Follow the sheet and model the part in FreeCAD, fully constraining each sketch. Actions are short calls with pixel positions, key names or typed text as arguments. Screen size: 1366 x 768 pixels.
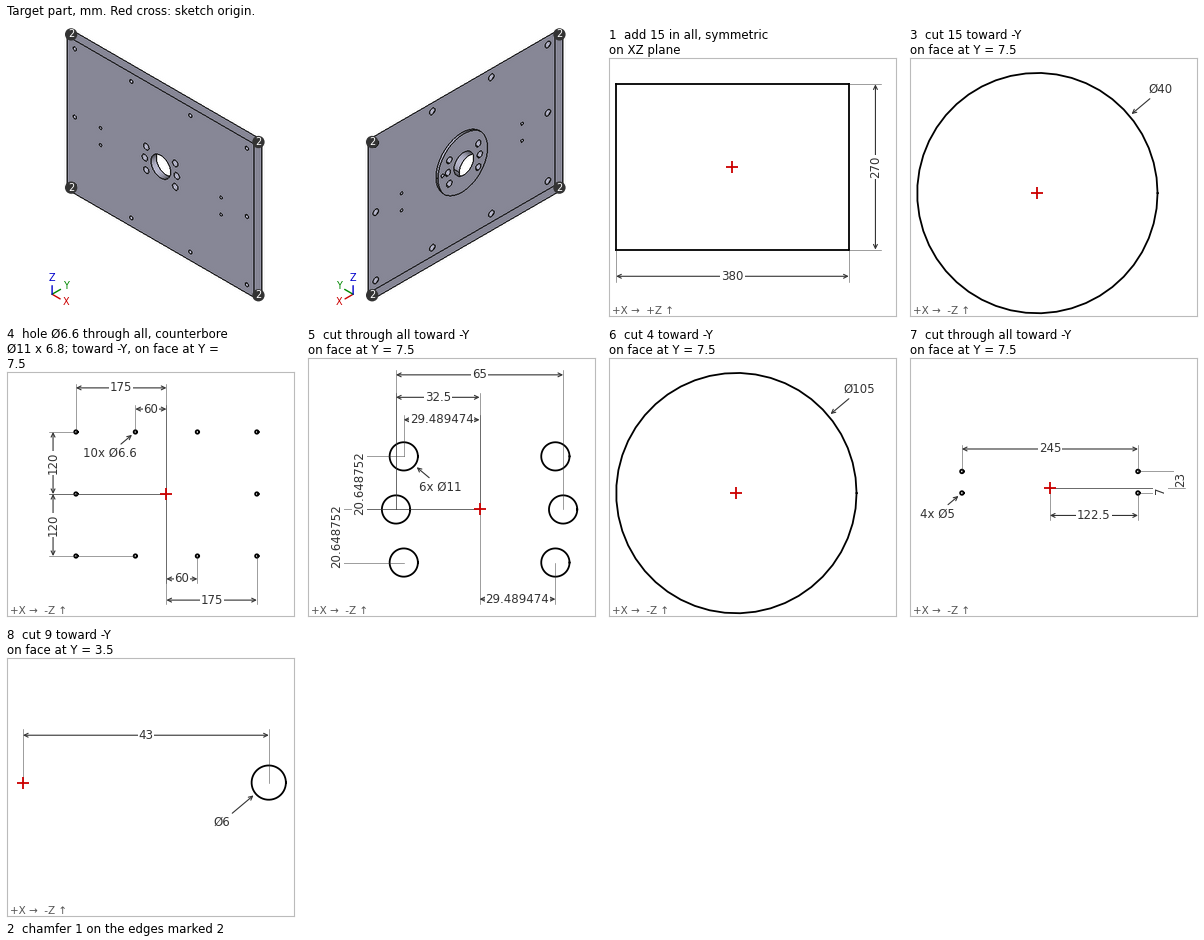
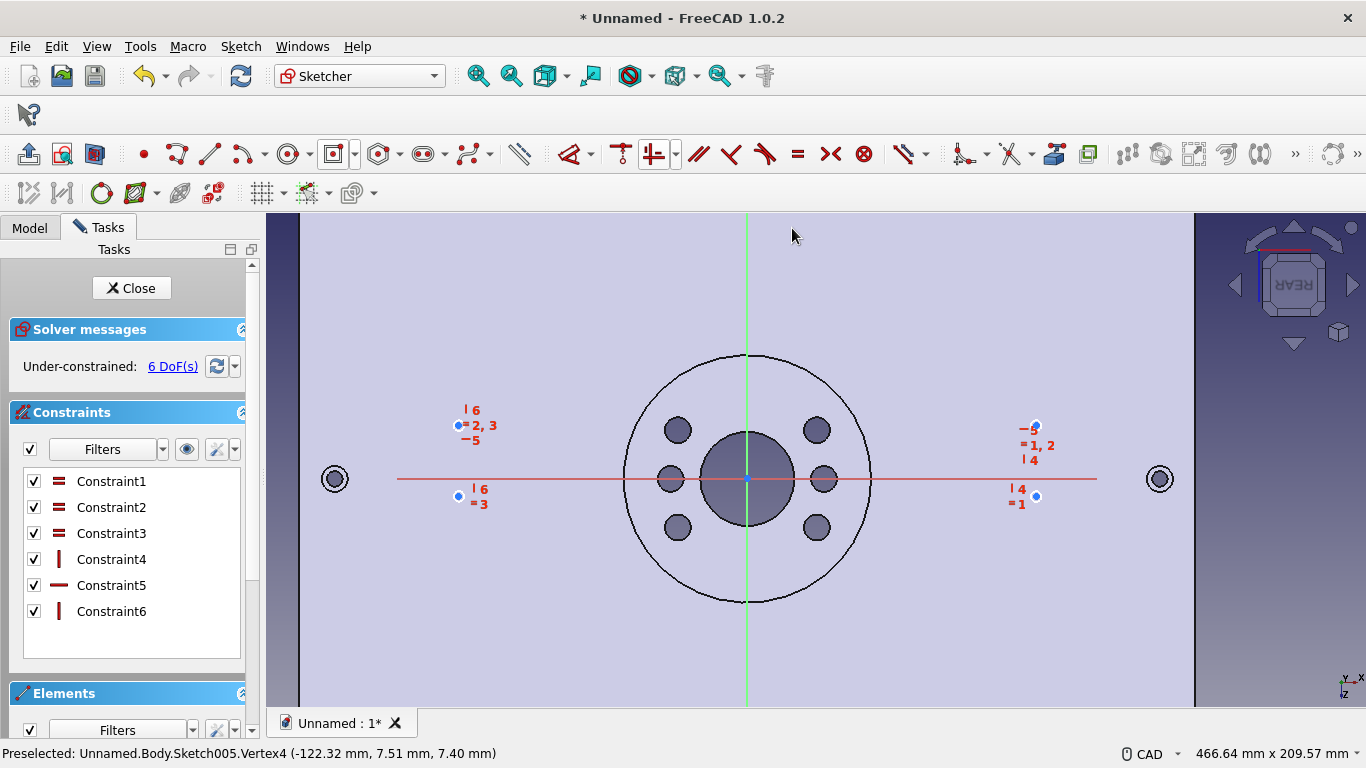
click(1036, 497)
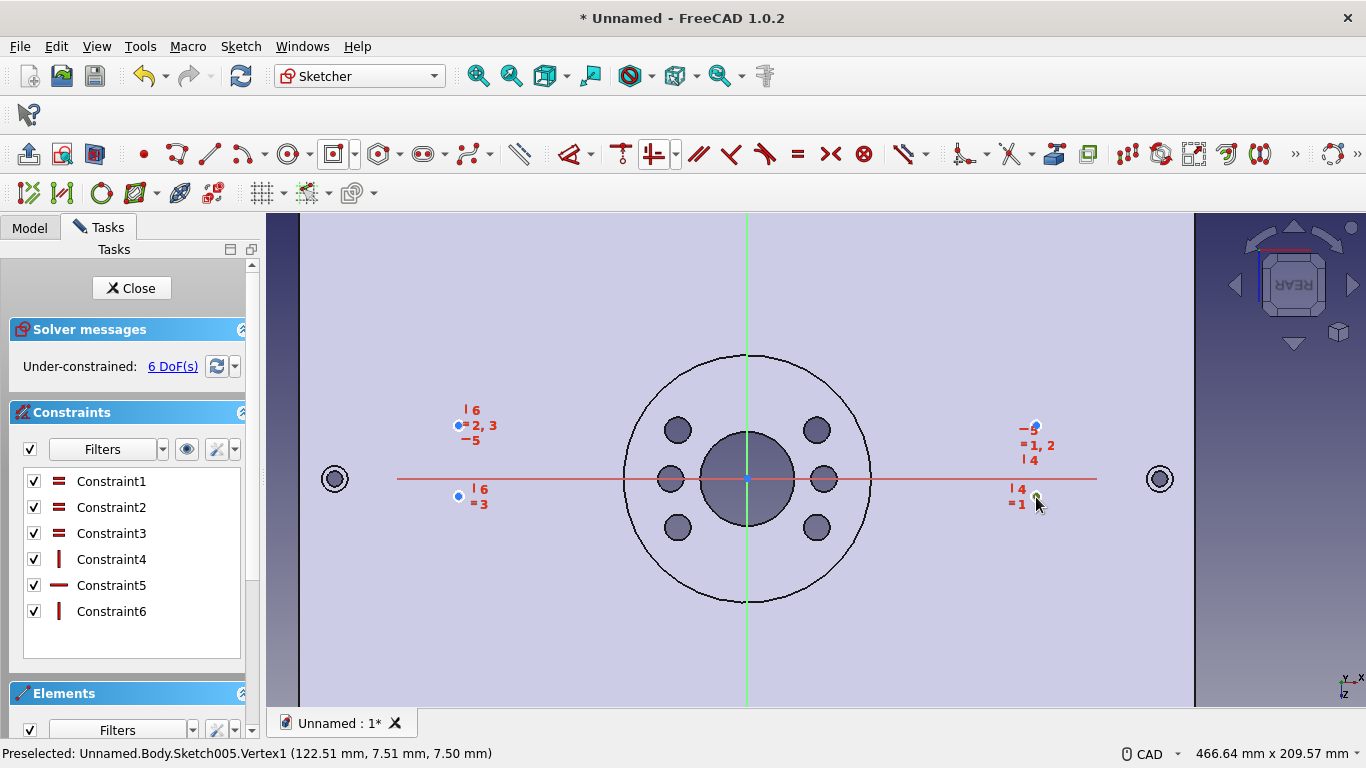
click(459, 496)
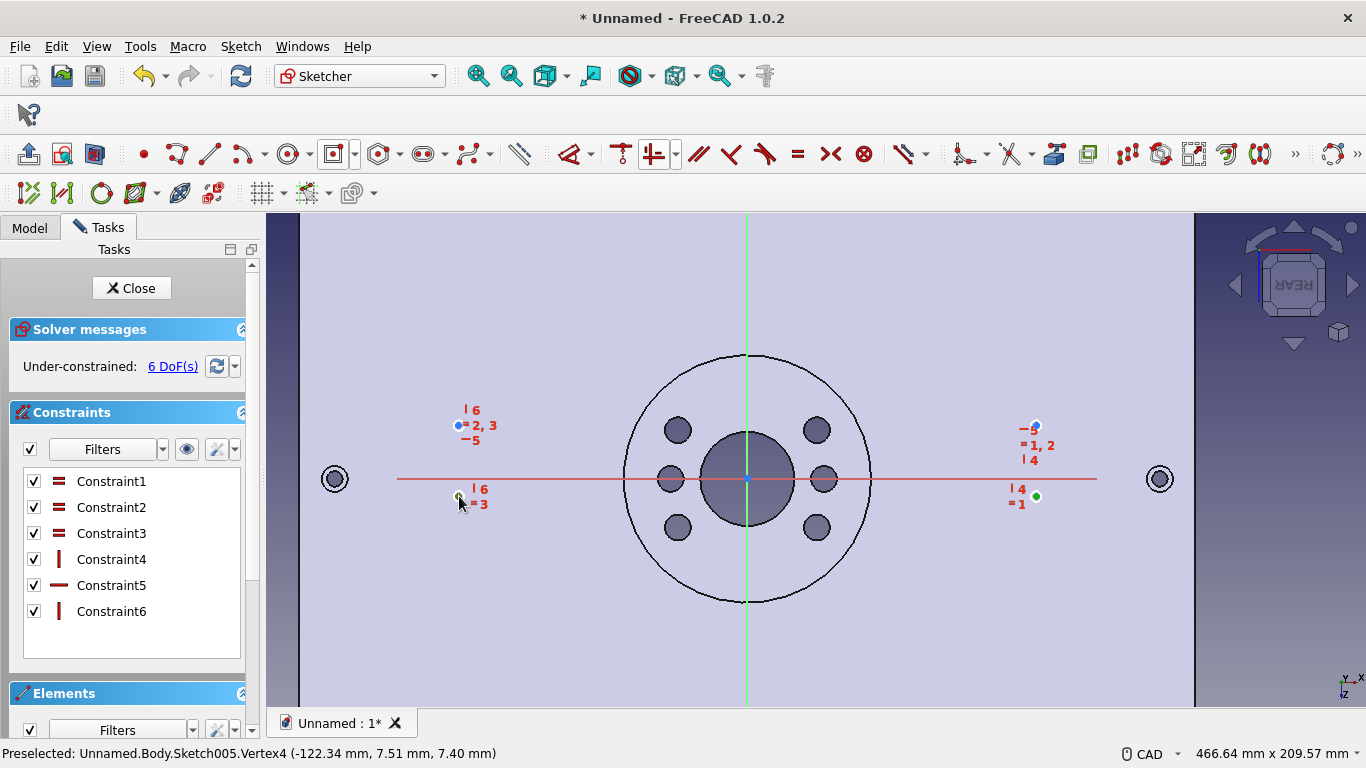
key(h)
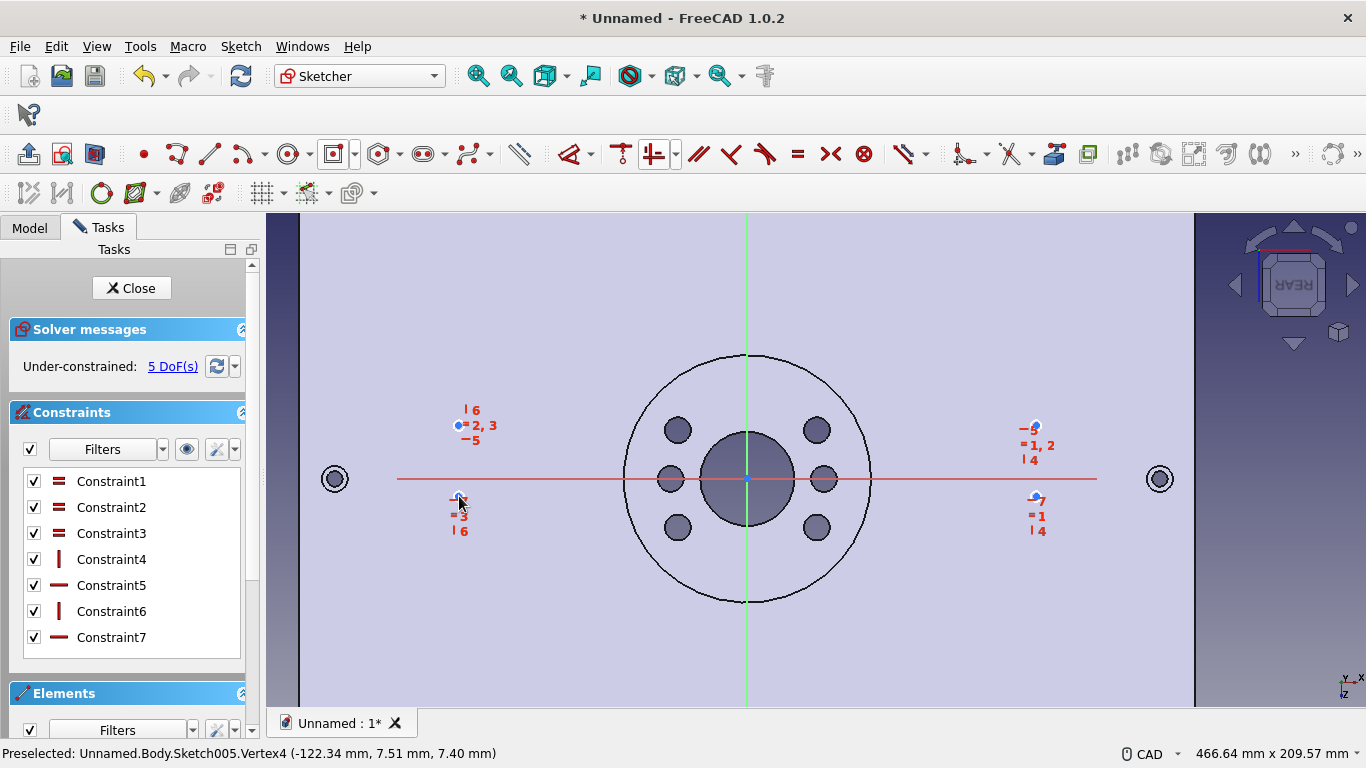
click(568, 154)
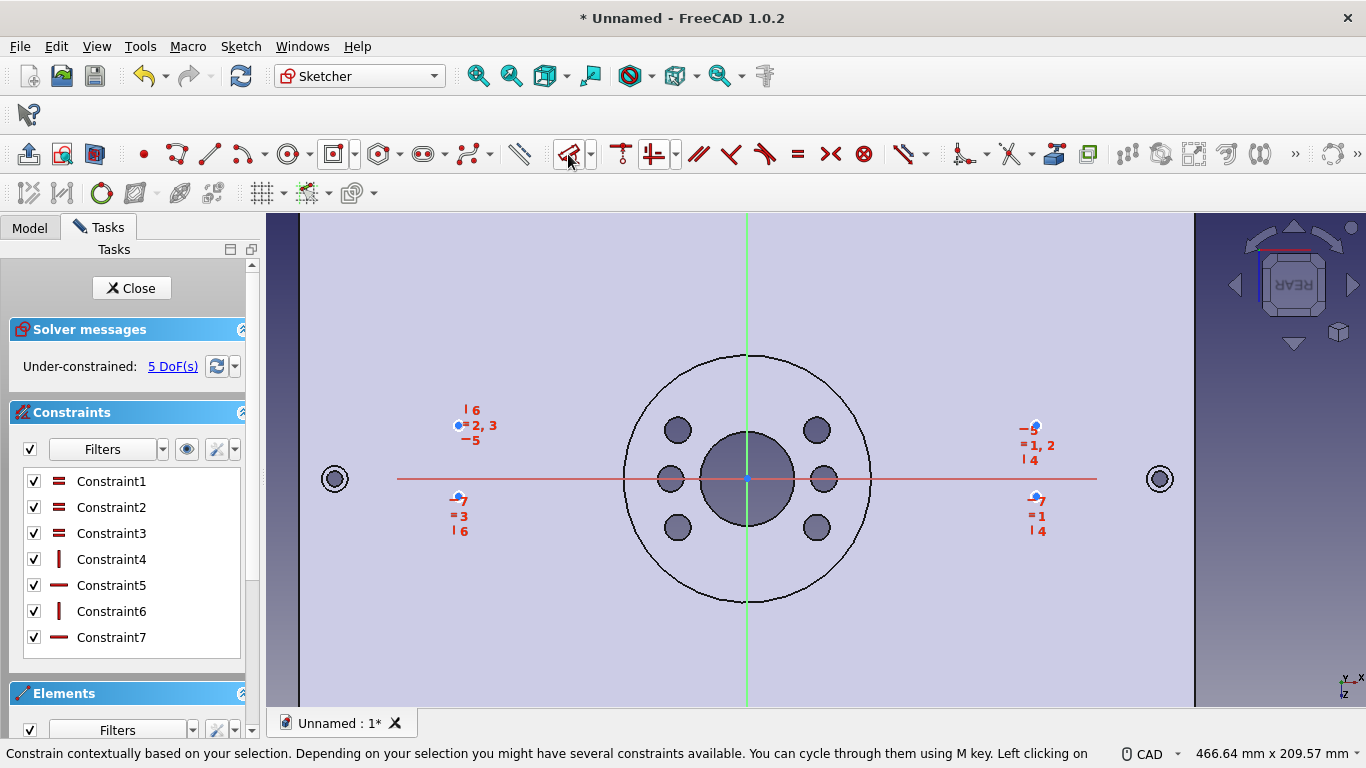
scroll(1032, 500, up, 7)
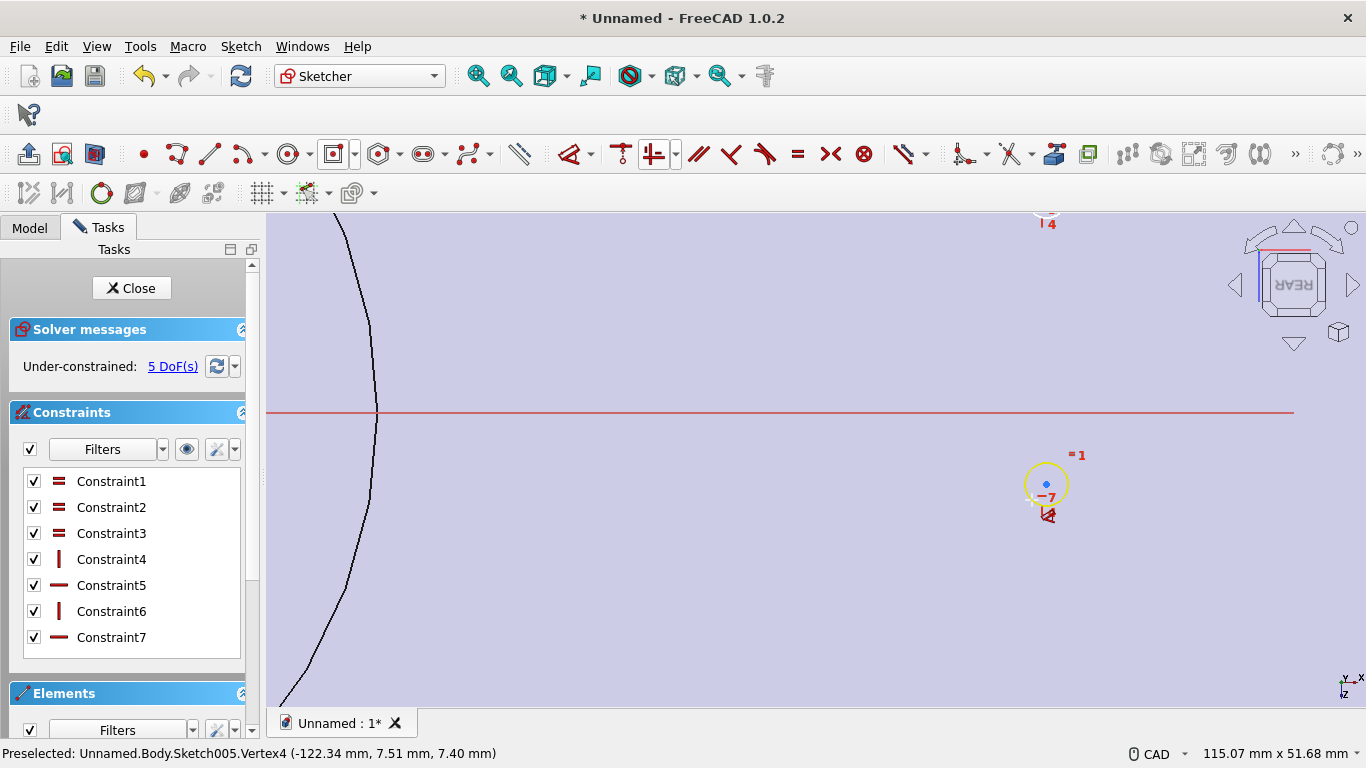
click(1032, 500)
click(1010, 523)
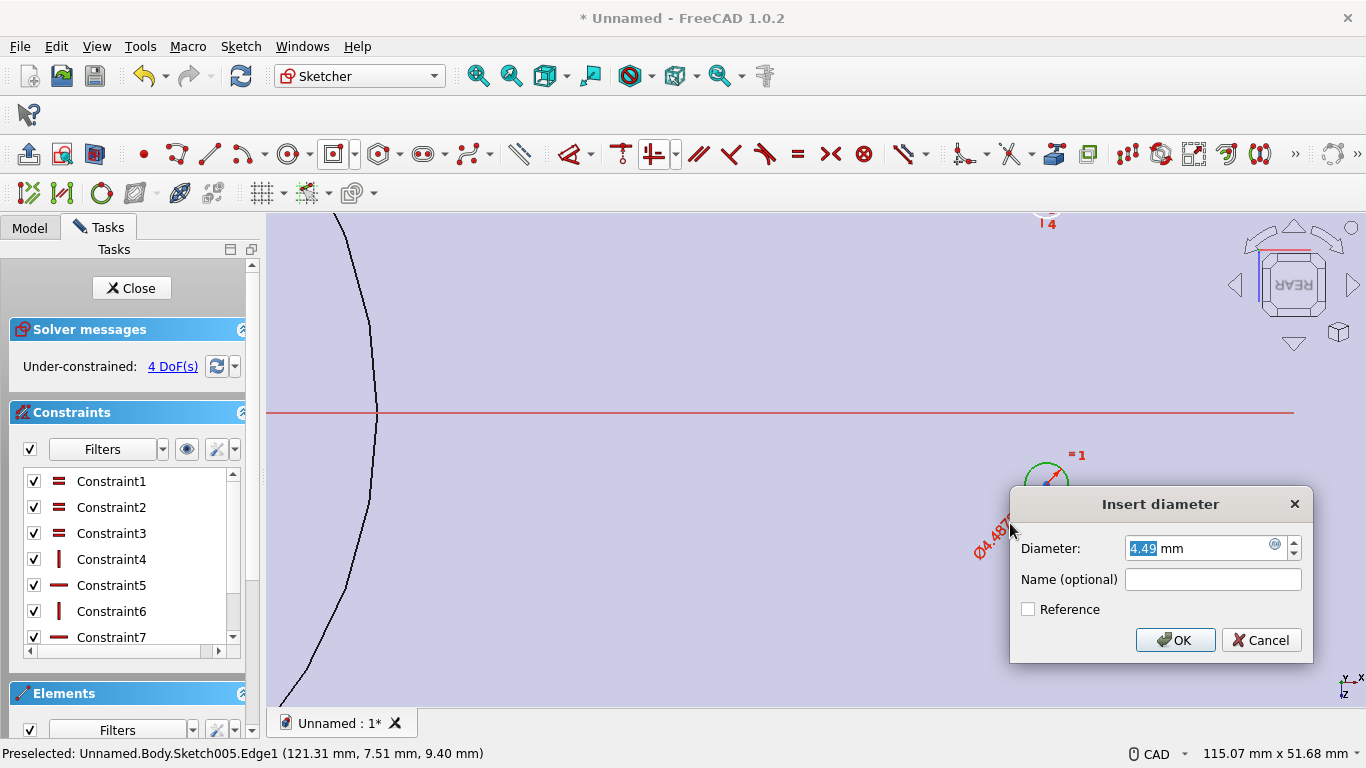
text(5)
key(Return)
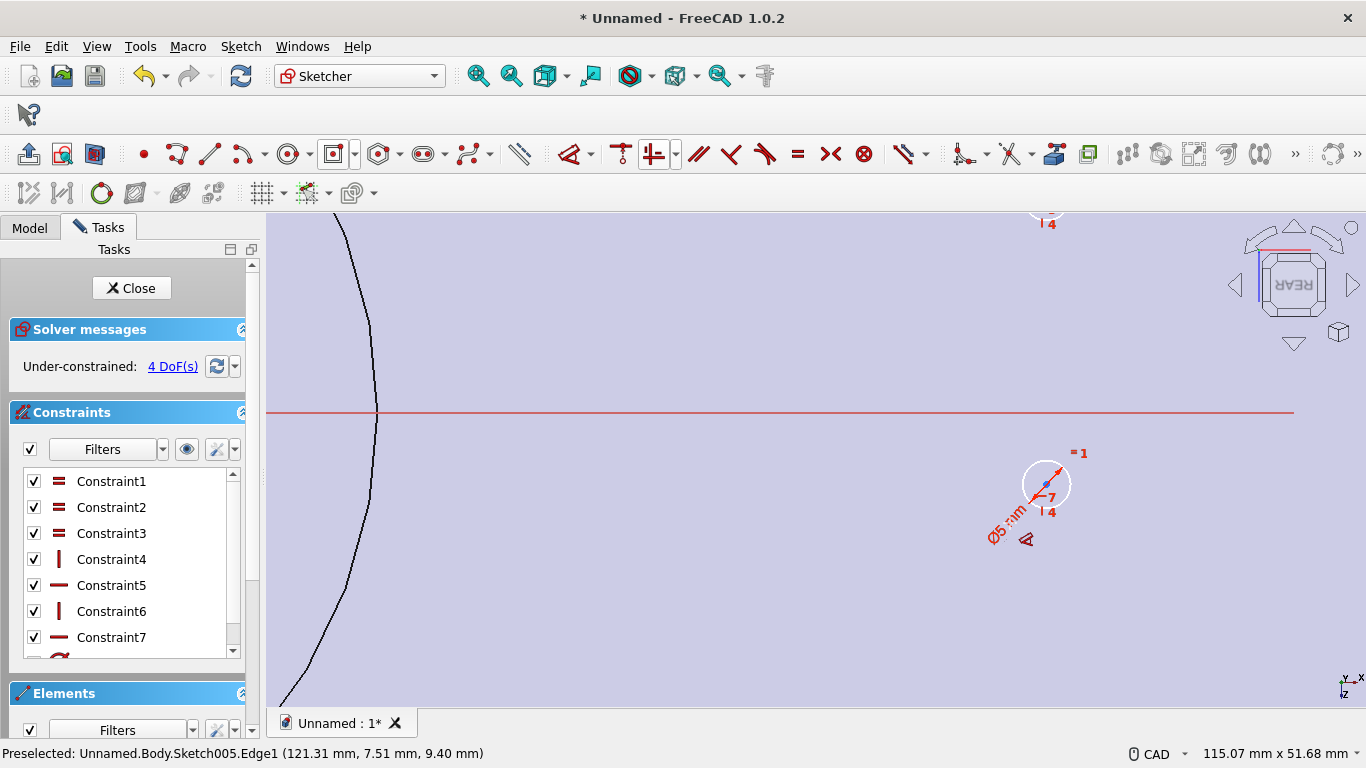
click(1047, 484)
click(1081, 449)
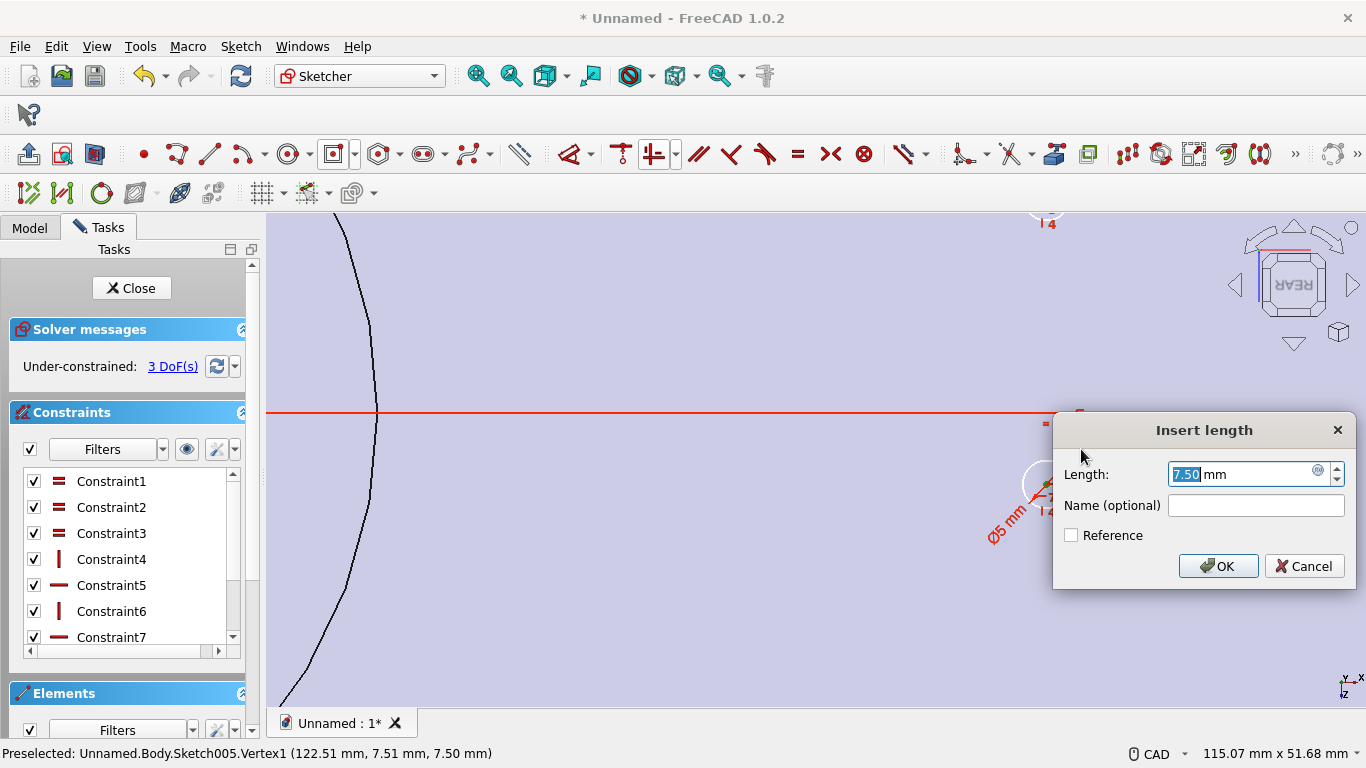
text(7)
key(Return)